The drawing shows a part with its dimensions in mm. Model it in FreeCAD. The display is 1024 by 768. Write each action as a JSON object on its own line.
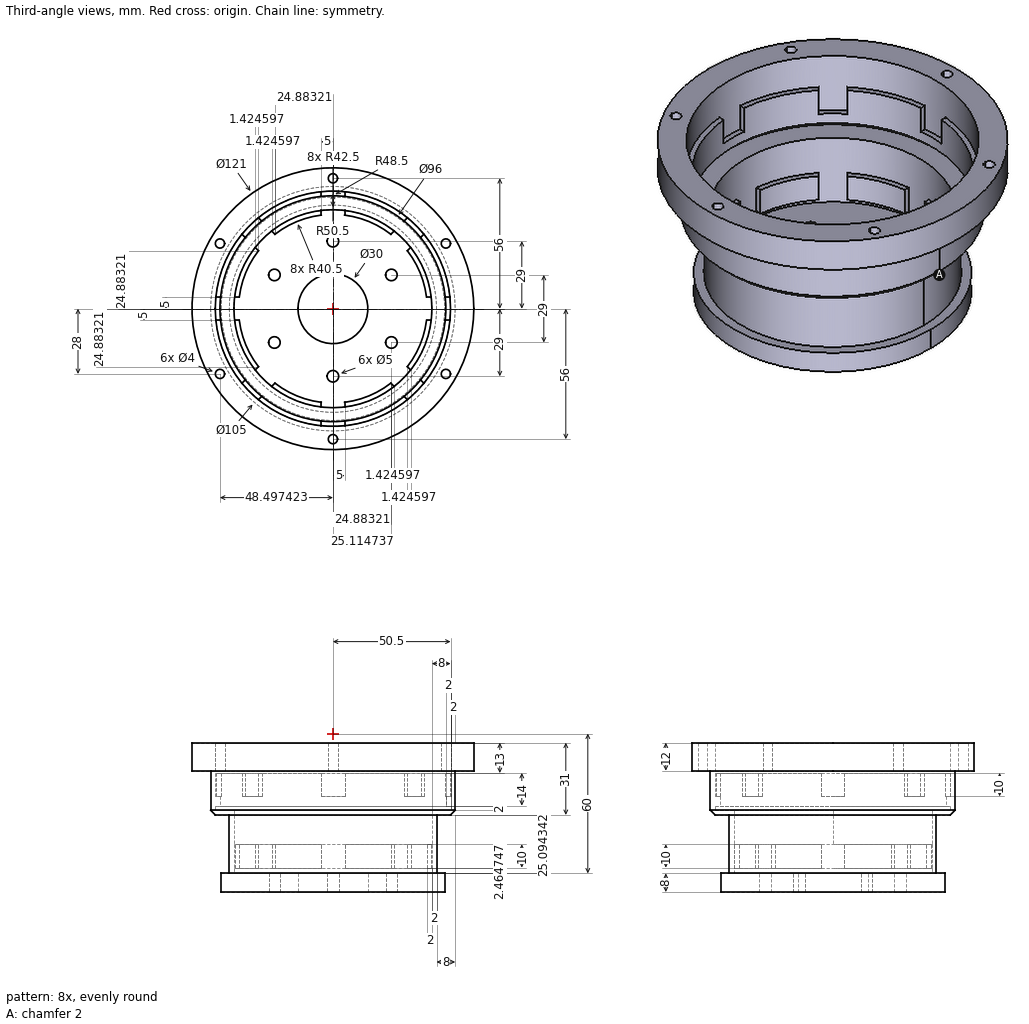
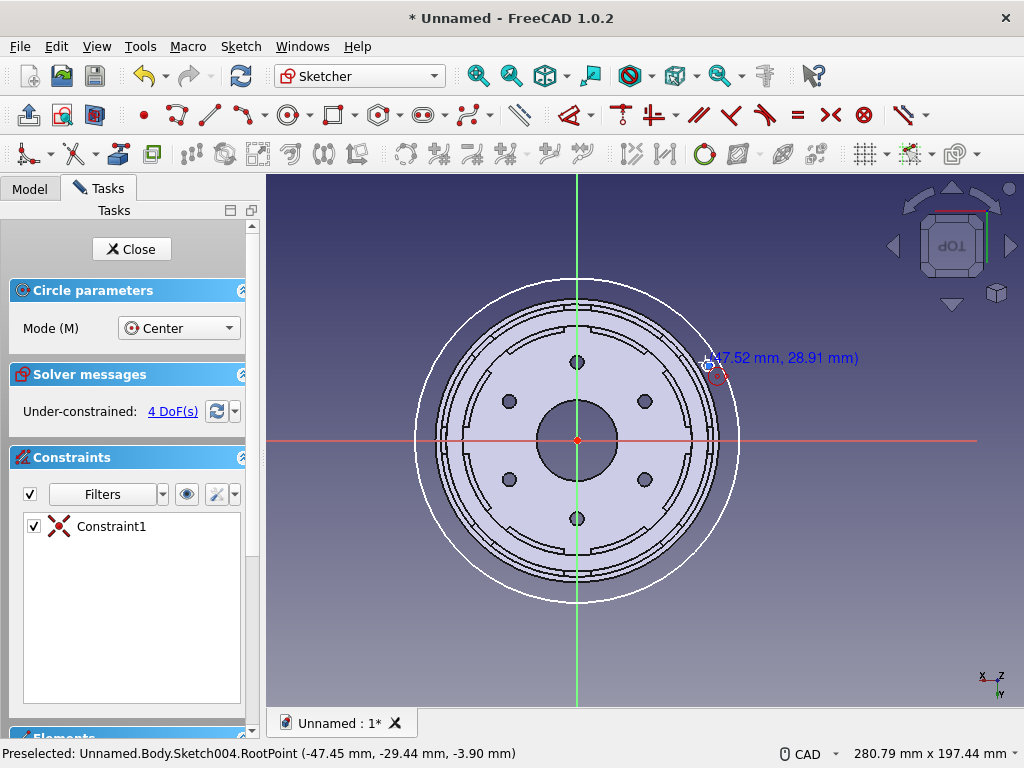
{"action": "scroll", "coordinate": [577, 289], "scroll_direction": "up", "scroll_amount": 8}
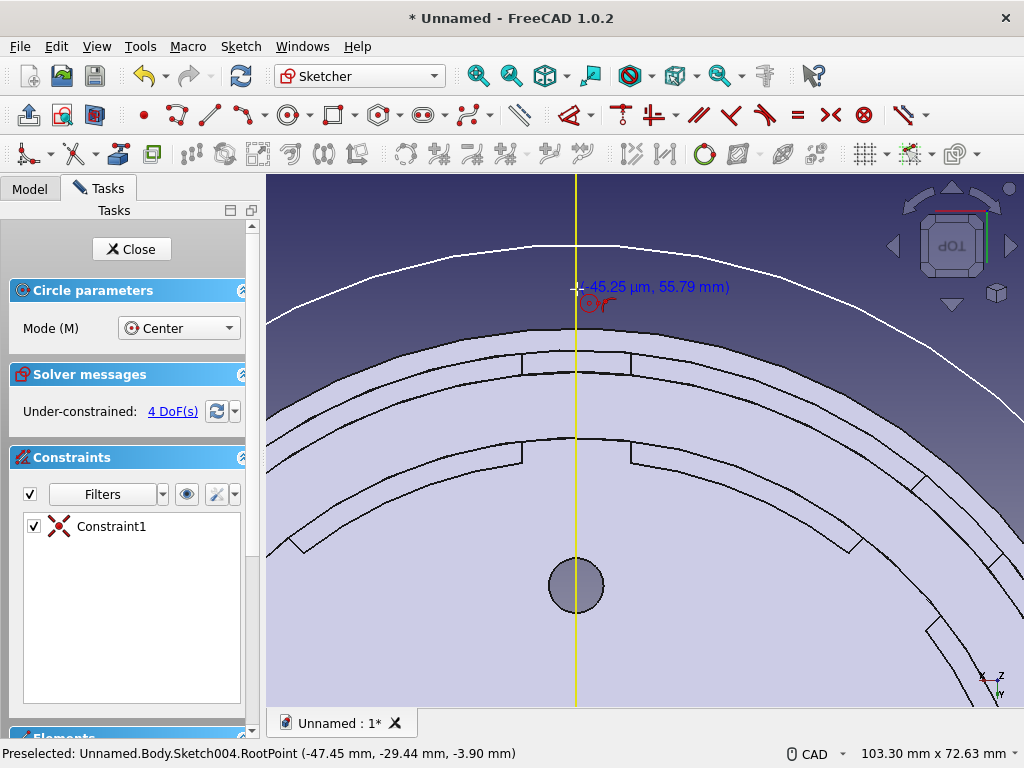
{"action": "scroll", "coordinate": [577, 289], "scroll_direction": "down", "scroll_amount": 8}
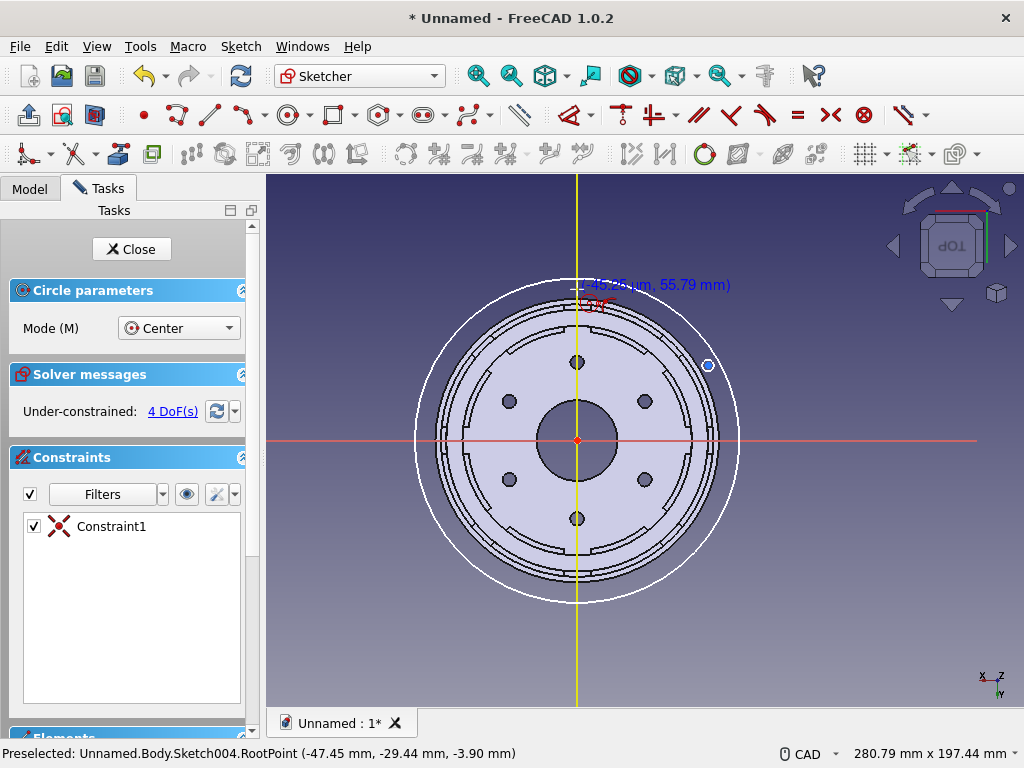
{"action": "scroll", "coordinate": [577, 289], "scroll_direction": "up", "scroll_amount": 2}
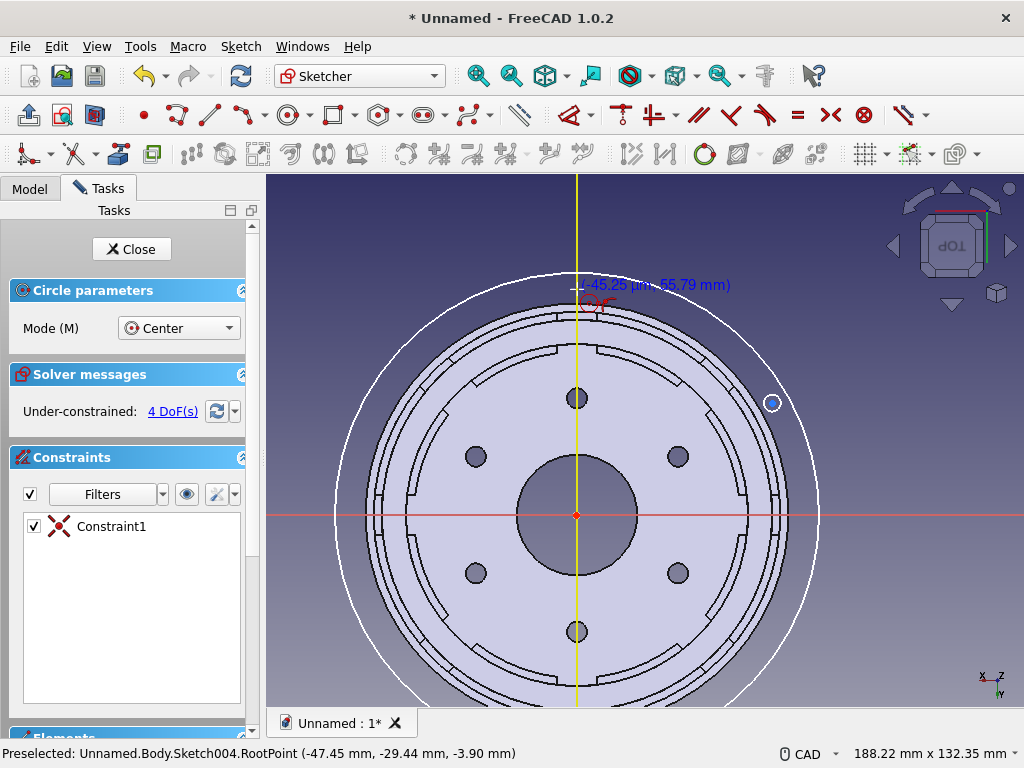
{"action": "left_click", "coordinate": [577, 290]}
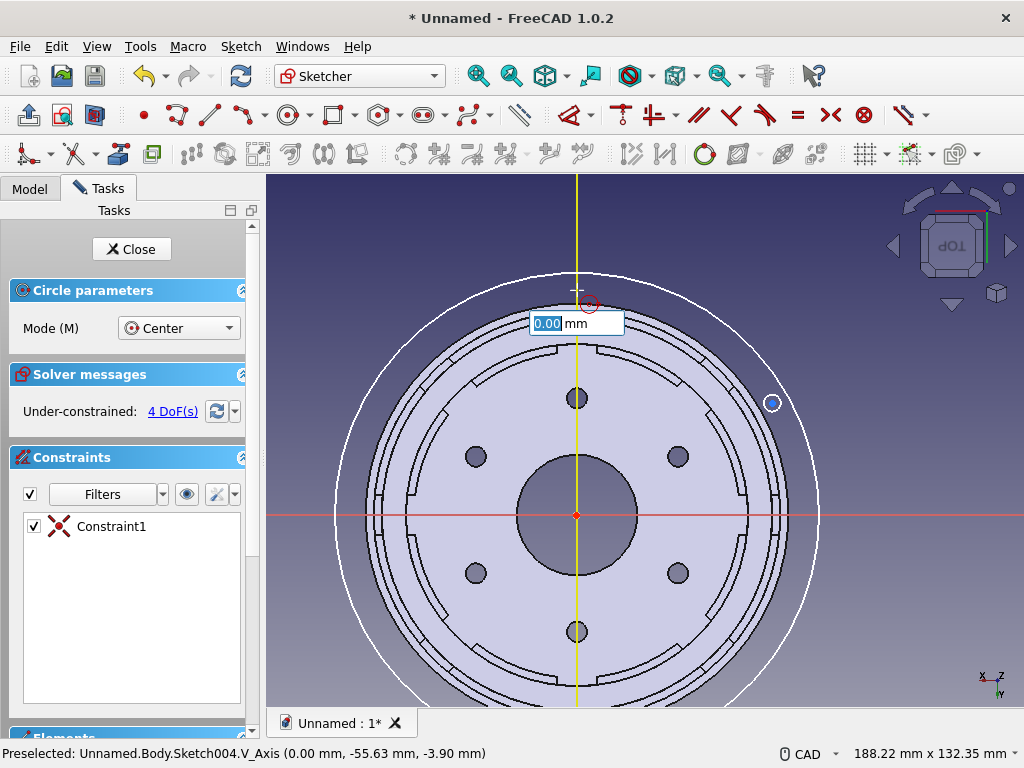
{"action": "scroll", "coordinate": [585, 287], "scroll_direction": "up", "scroll_amount": 4}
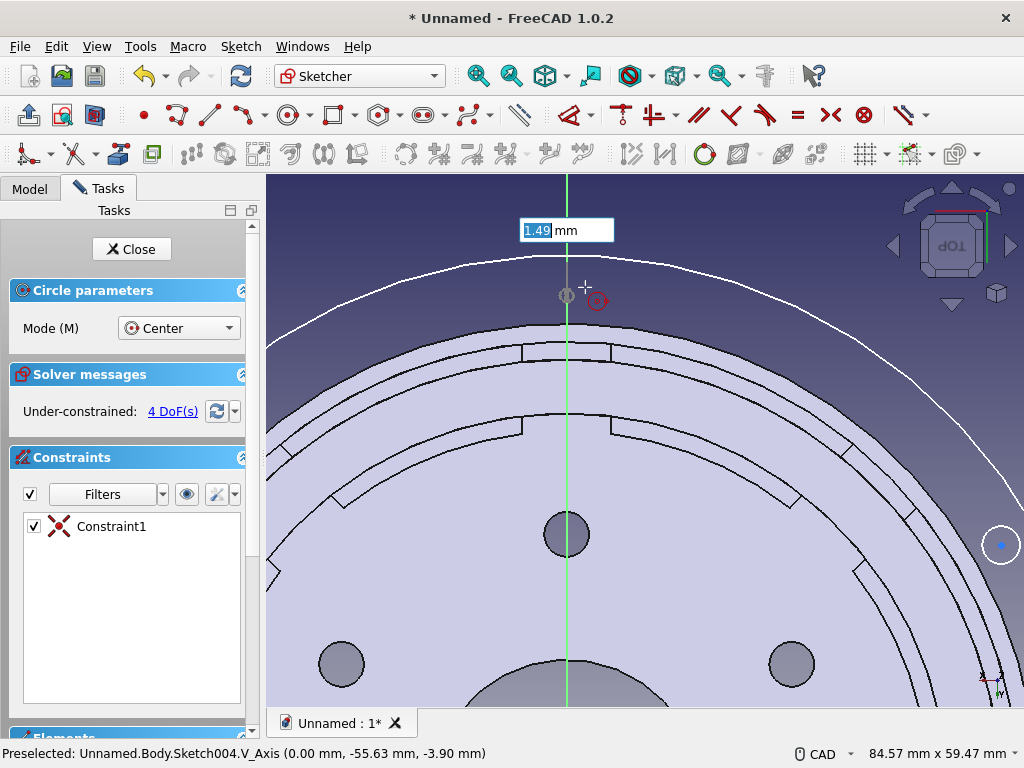
{"action": "left_click", "coordinate": [583, 286]}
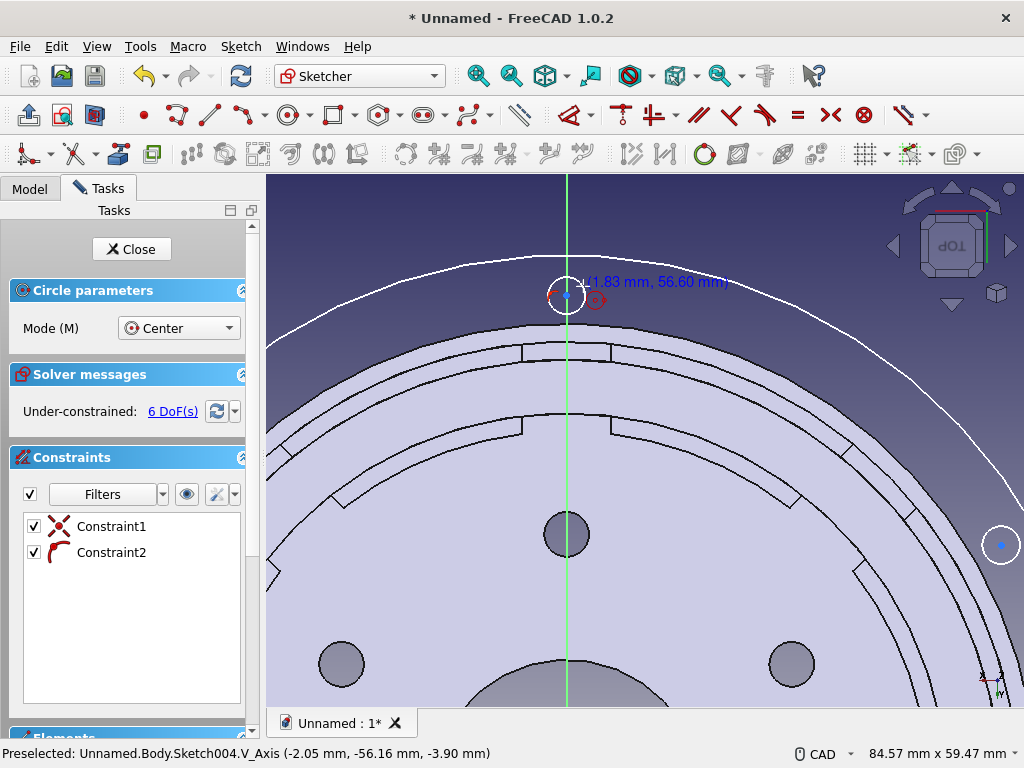
{"action": "scroll", "coordinate": [581, 288], "scroll_direction": "down", "scroll_amount": 6}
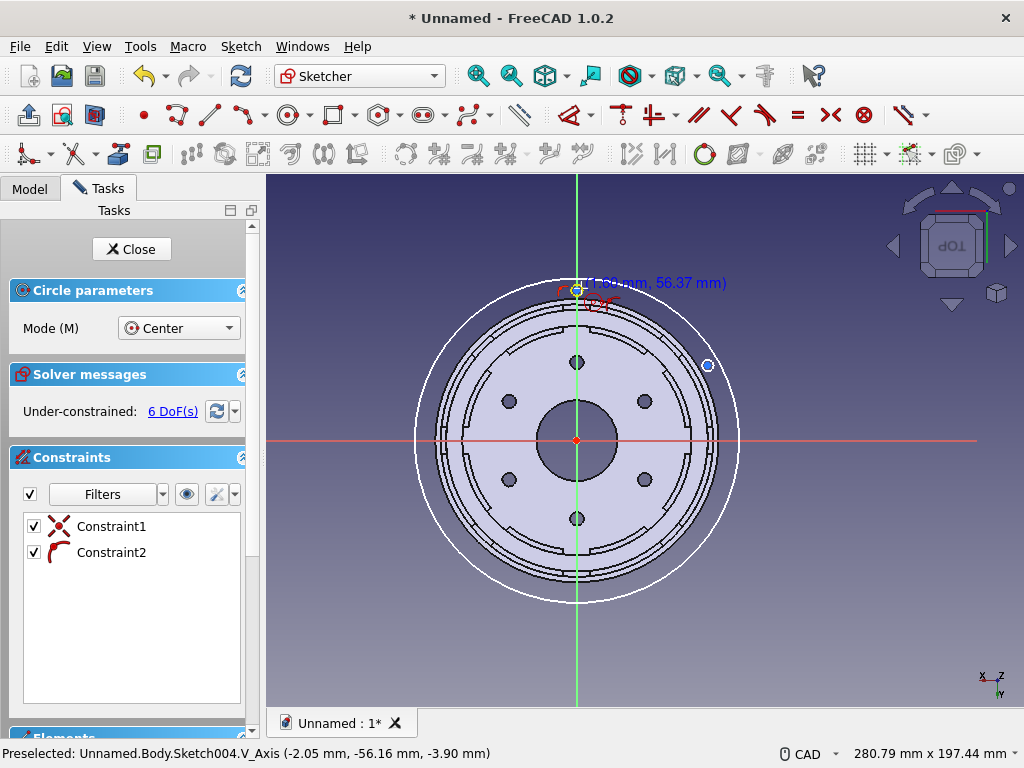
{"action": "scroll", "coordinate": [446, 365], "scroll_direction": "up", "scroll_amount": 8}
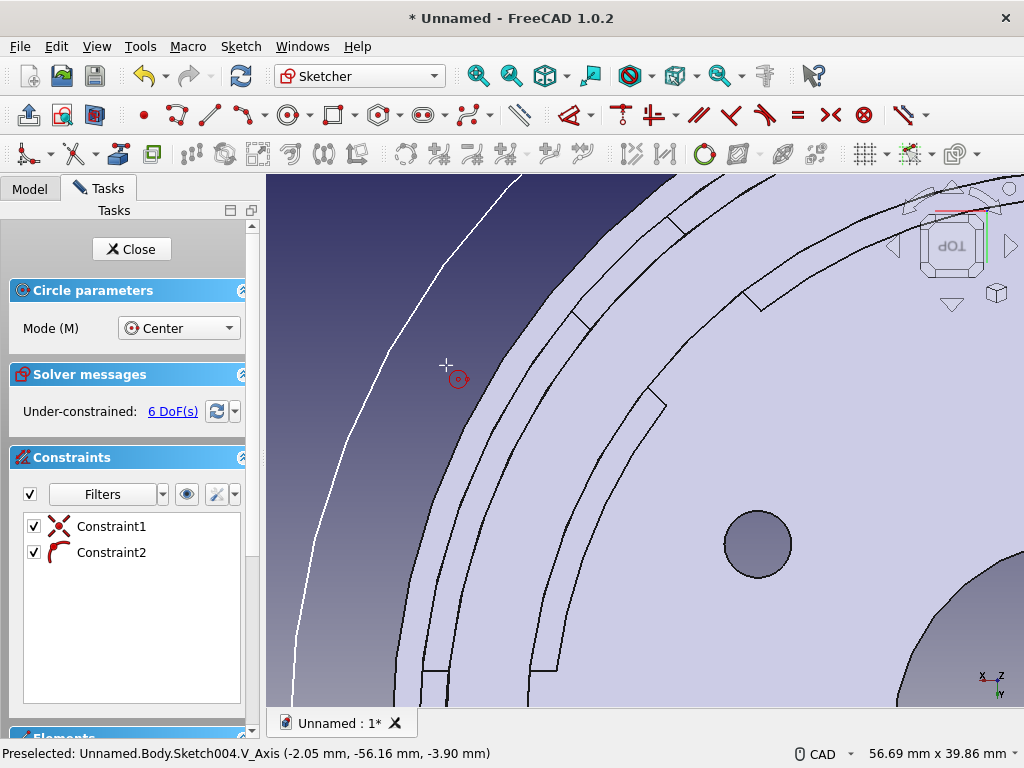
{"action": "scroll", "coordinate": [446, 365], "scroll_direction": "down", "scroll_amount": 8}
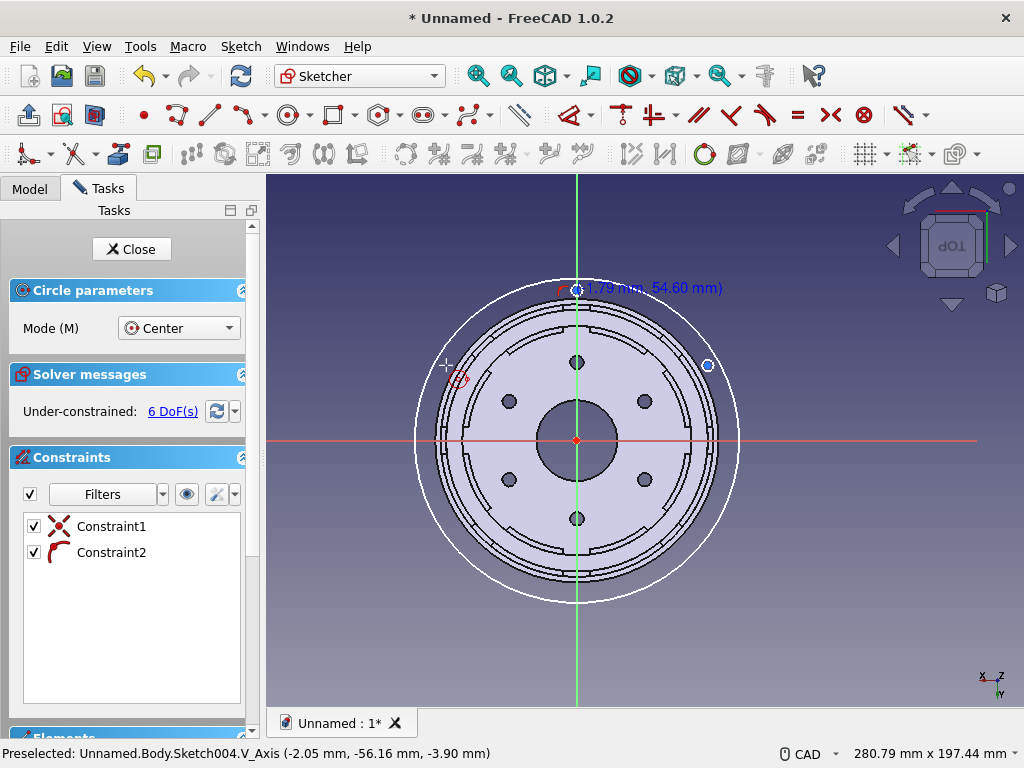
{"action": "scroll", "coordinate": [446, 365], "scroll_direction": "up", "scroll_amount": 2}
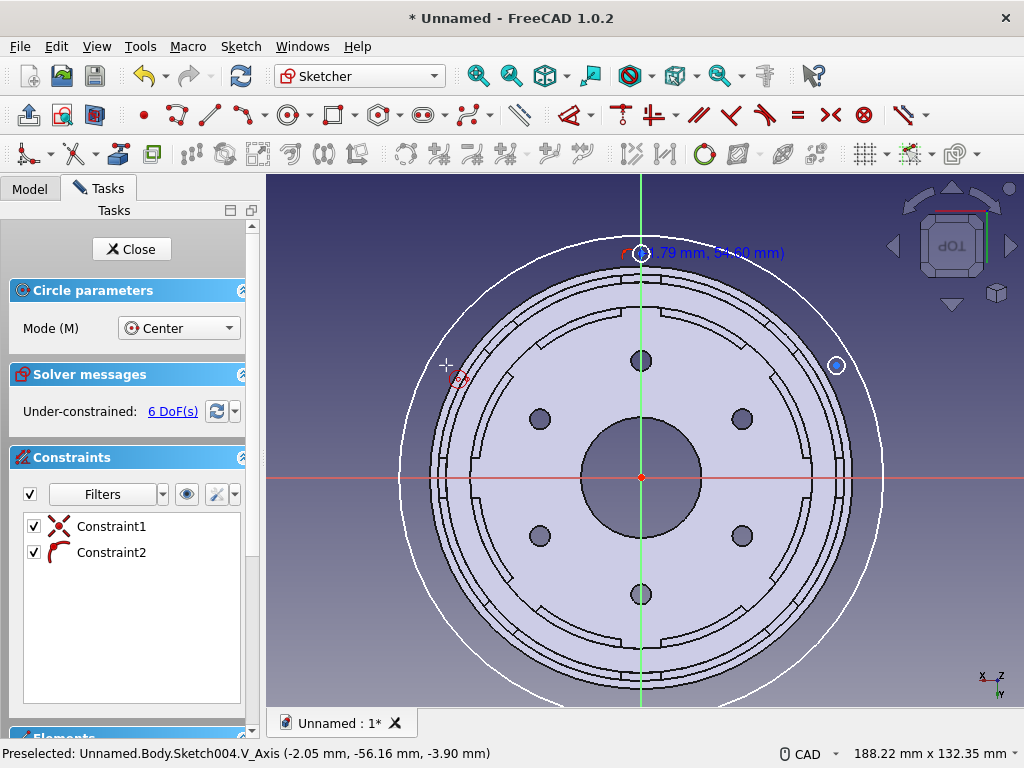
{"action": "left_click", "coordinate": [446, 365]}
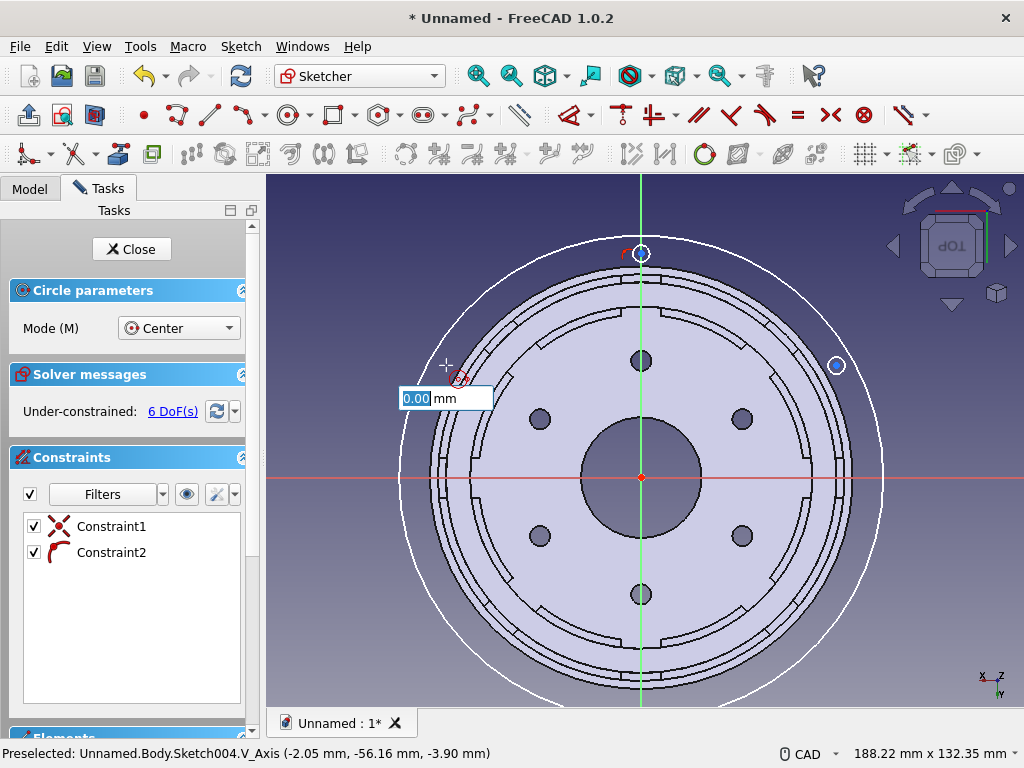
{"action": "scroll", "coordinate": [452, 359], "scroll_direction": "up", "scroll_amount": 4}